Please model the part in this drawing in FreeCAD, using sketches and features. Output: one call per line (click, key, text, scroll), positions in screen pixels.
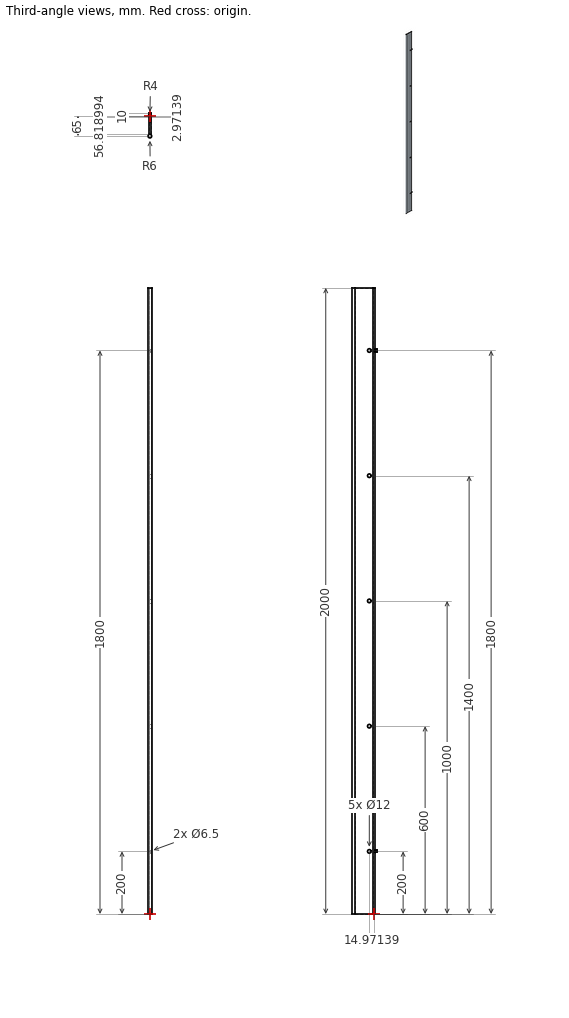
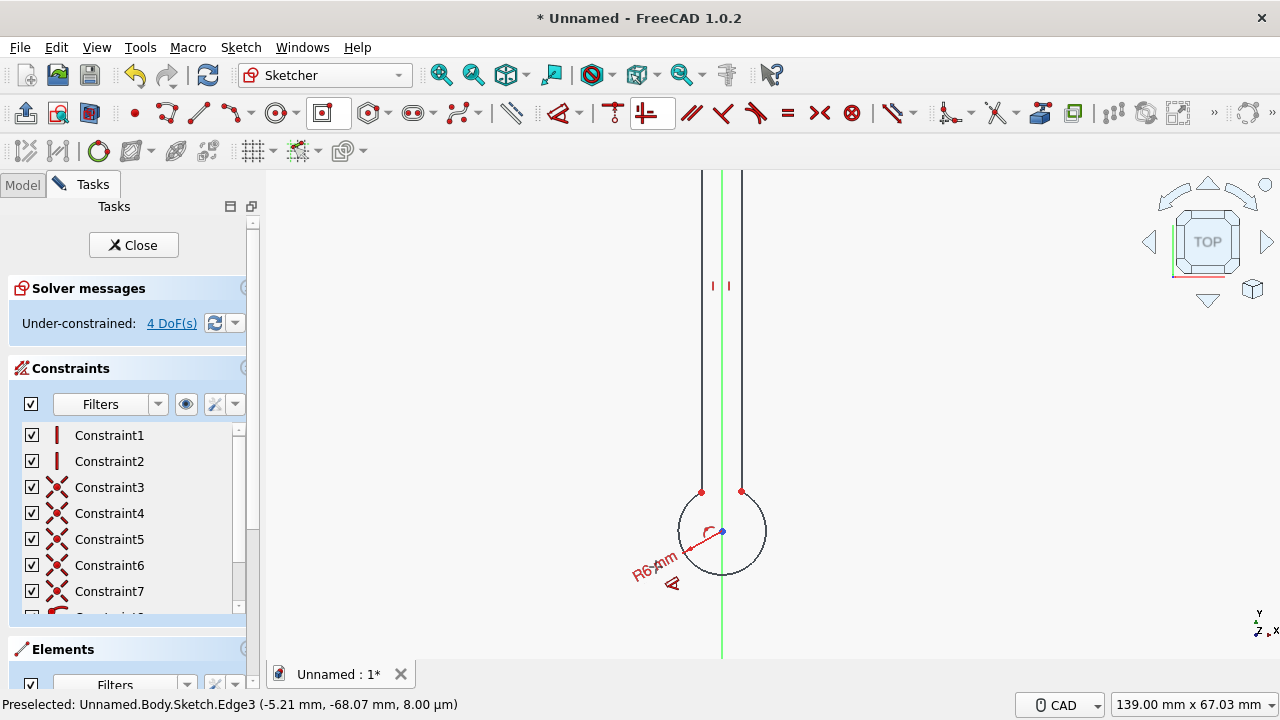
scroll(683, 553, down, 3)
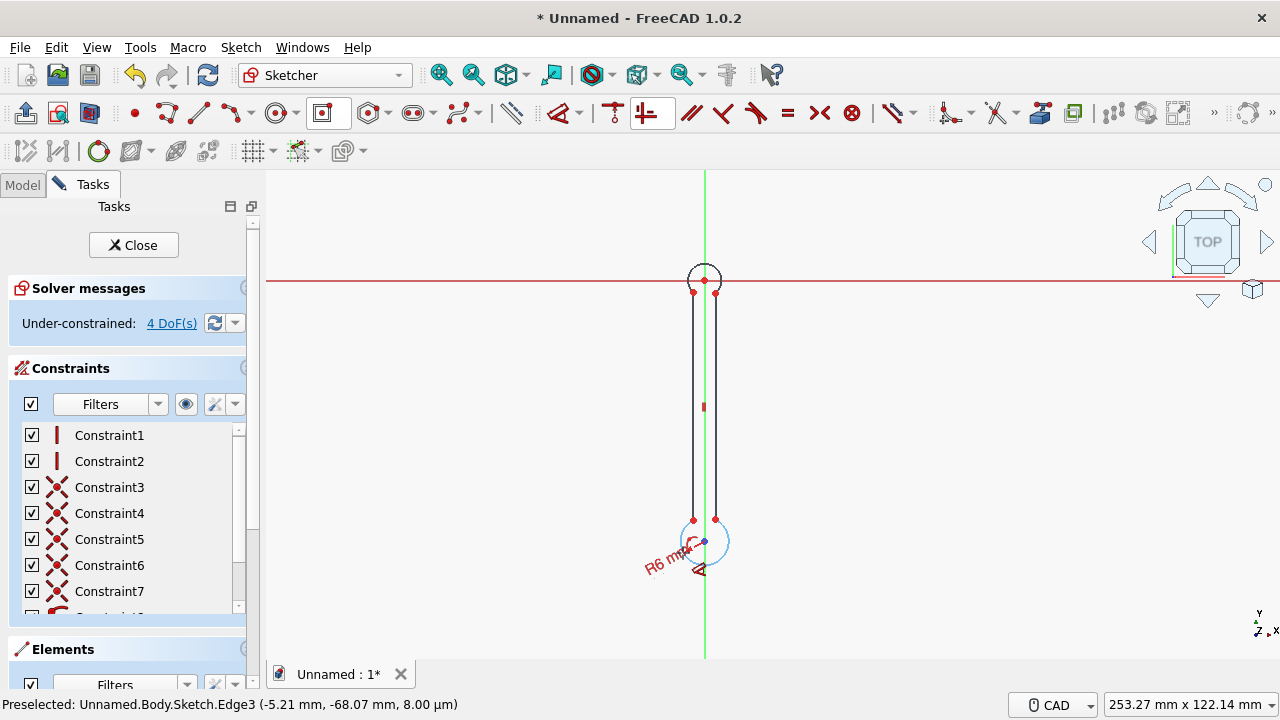
scroll(719, 271, up, 5)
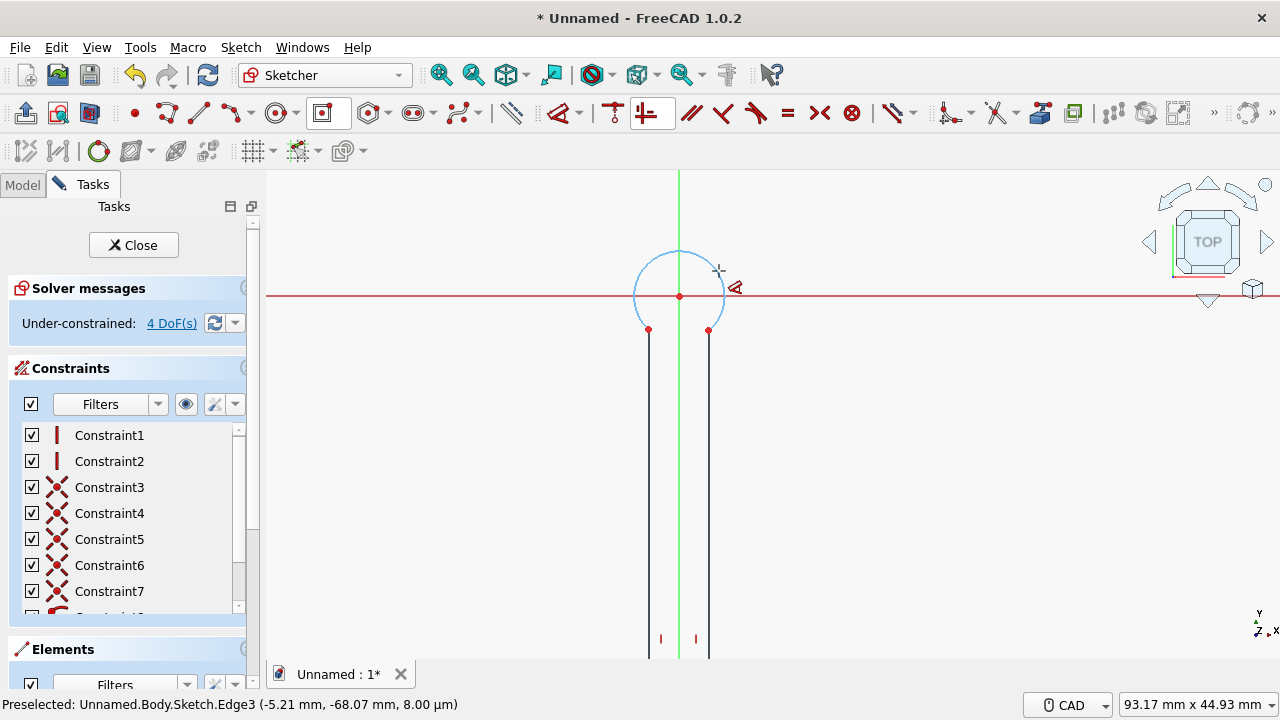
click(717, 271)
click(743, 253)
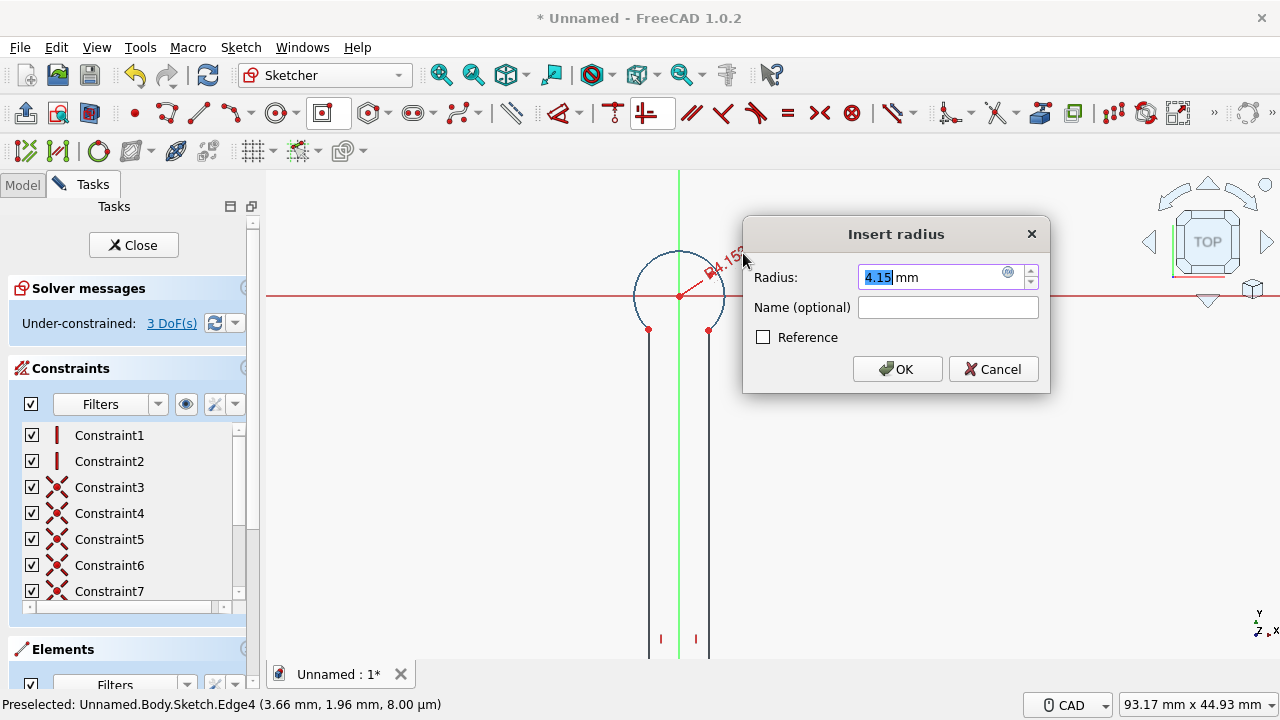
text(4)
key(Return)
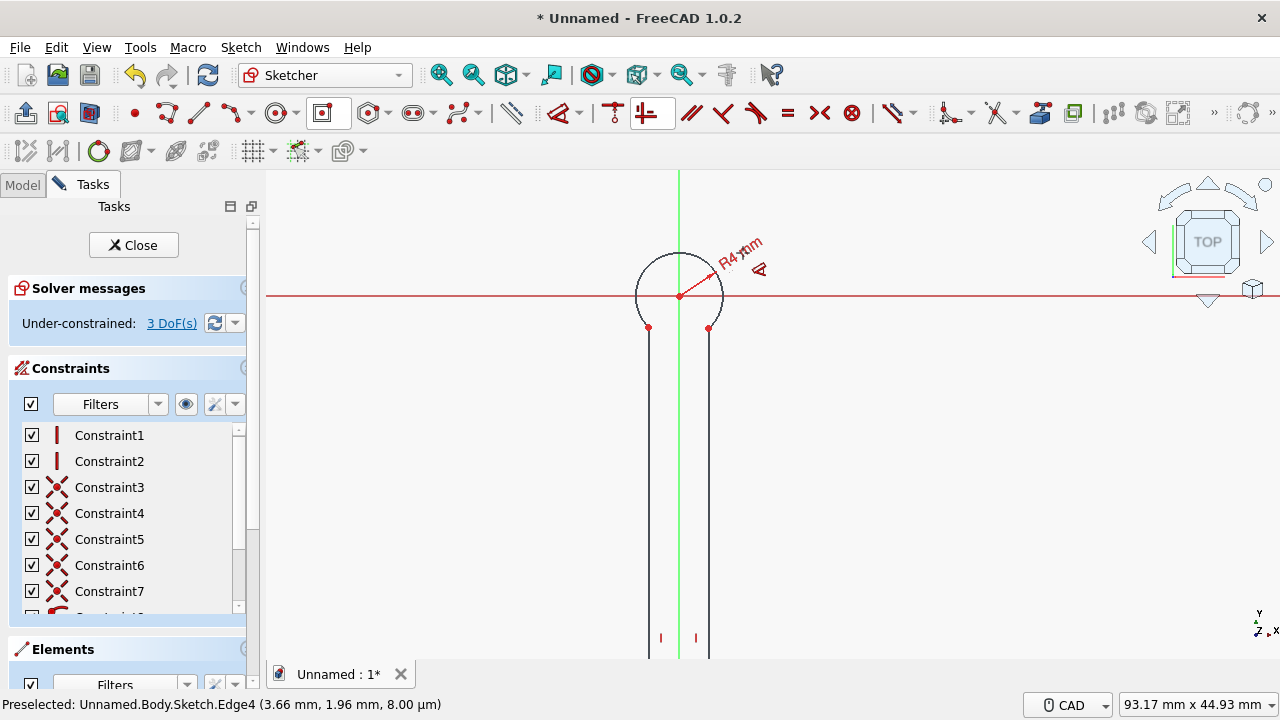
scroll(719, 271, down, 5)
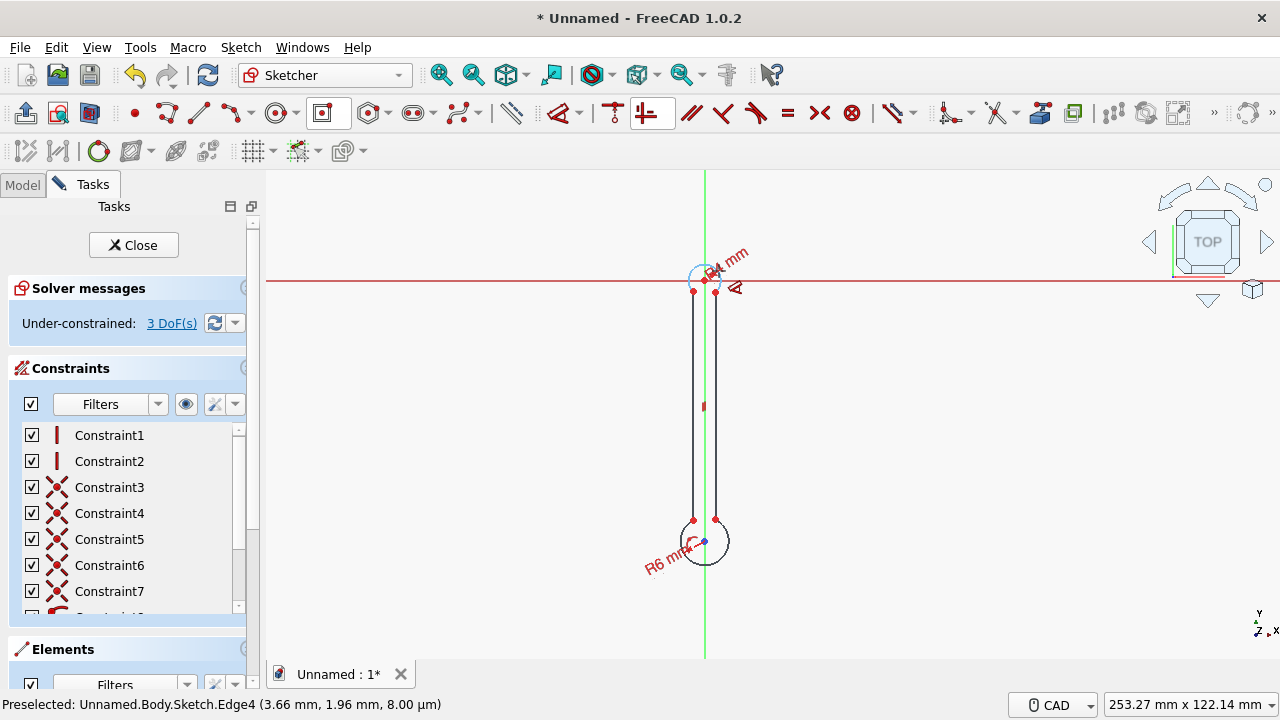
click(705, 541)
click(739, 411)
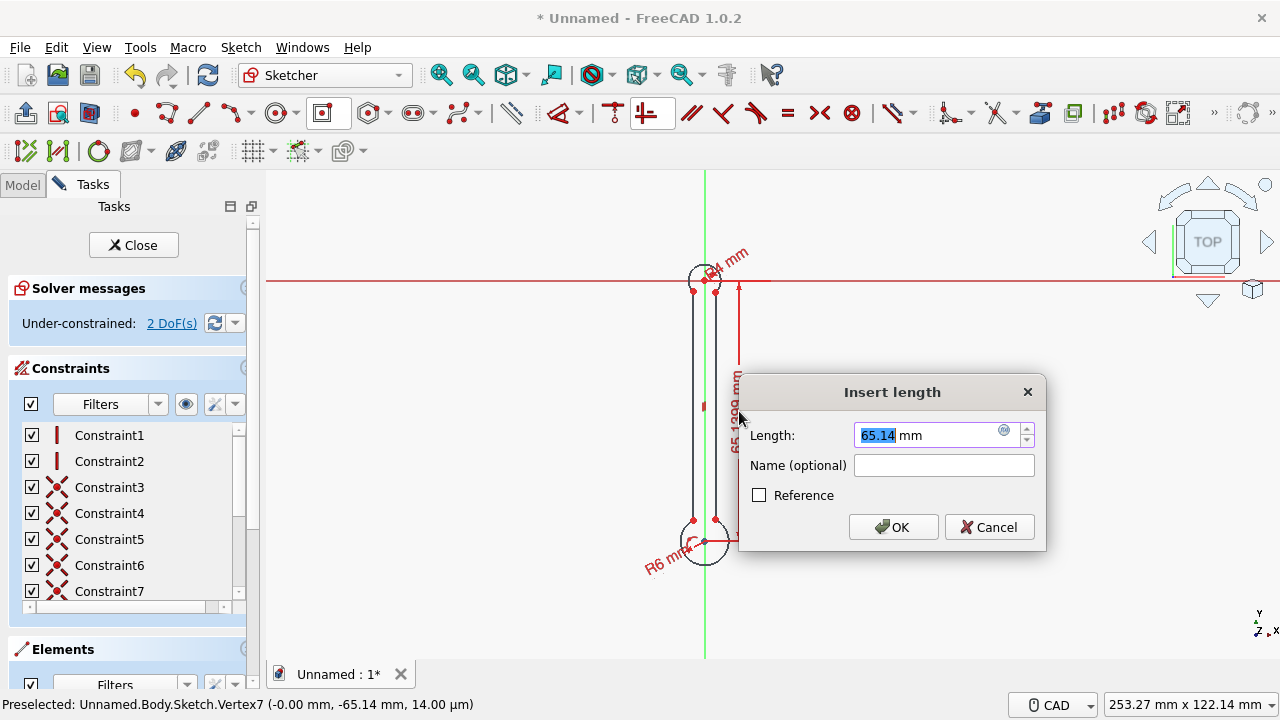
text(65)
key(Return)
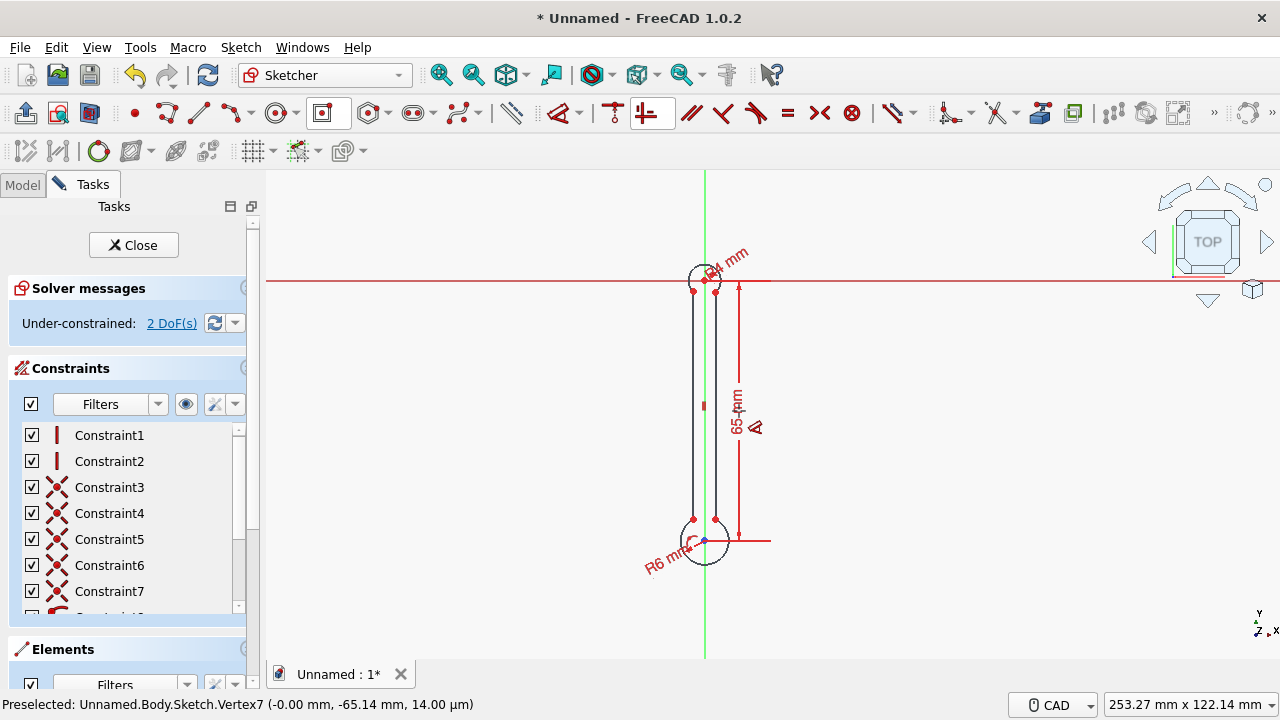
scroll(716, 292, up, 7)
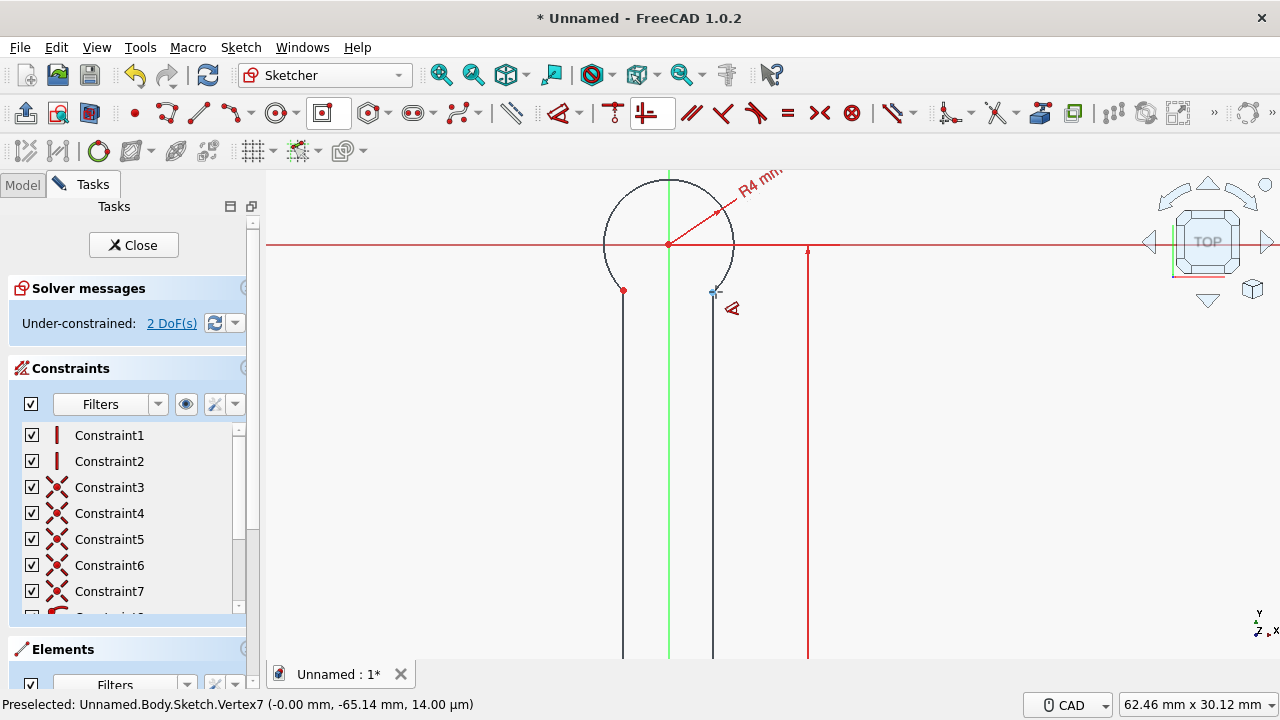
click(713, 292)
click(747, 269)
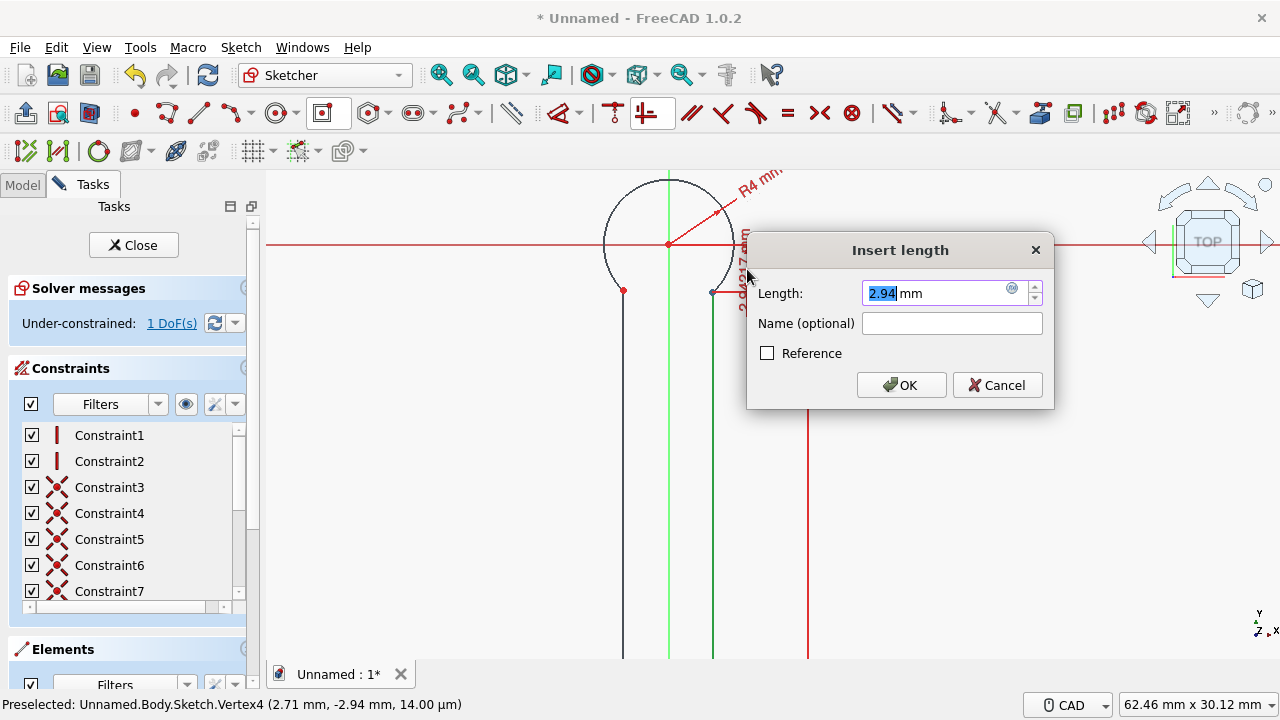
text(2.97139)
key(Return)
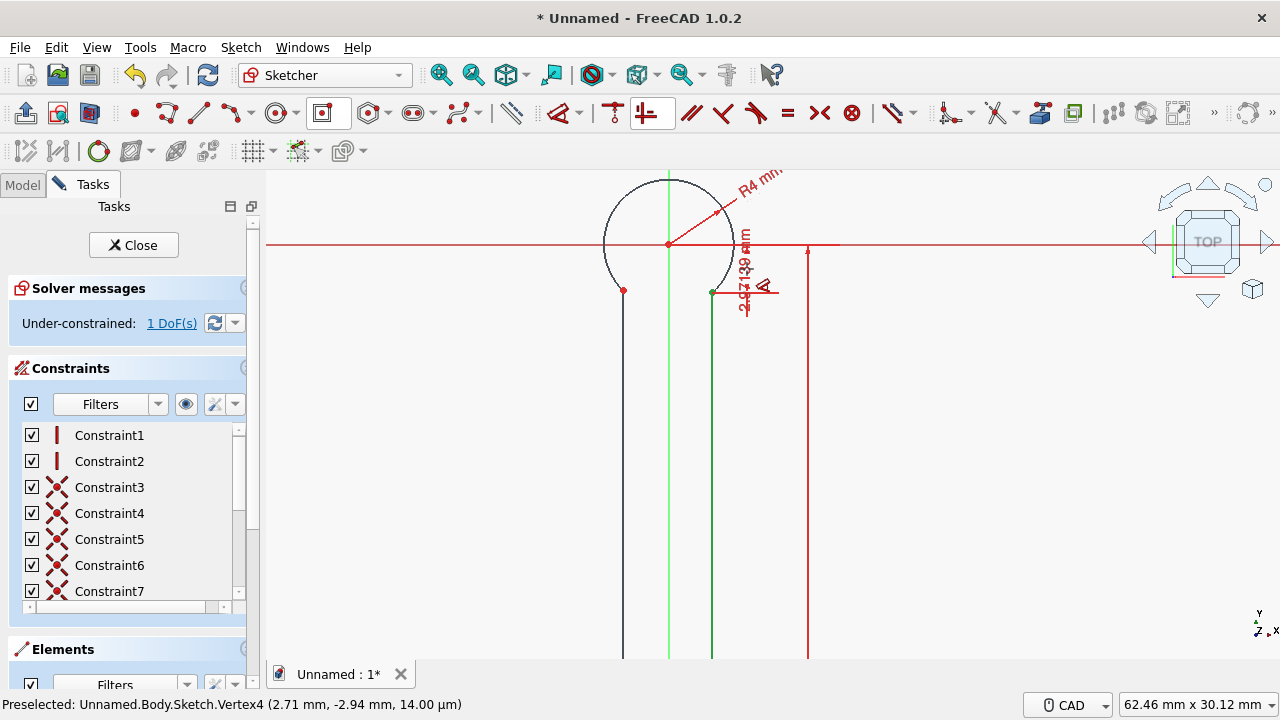
scroll(716, 292, down, 7)